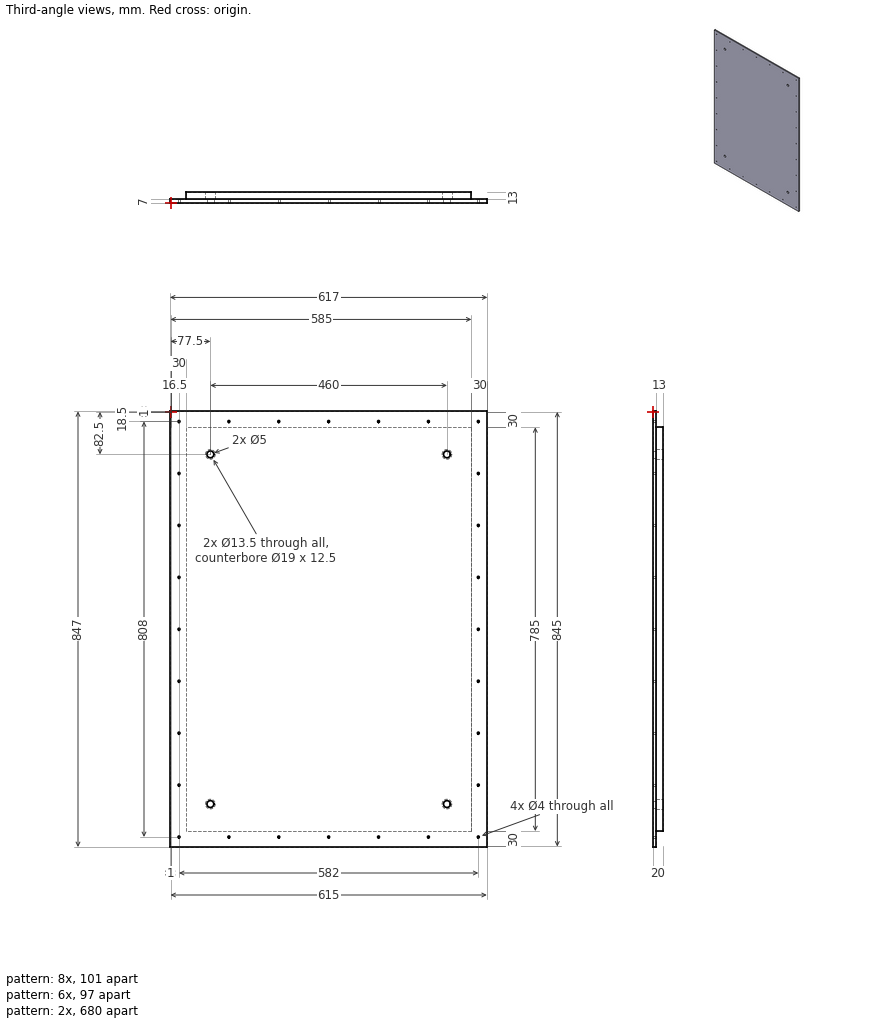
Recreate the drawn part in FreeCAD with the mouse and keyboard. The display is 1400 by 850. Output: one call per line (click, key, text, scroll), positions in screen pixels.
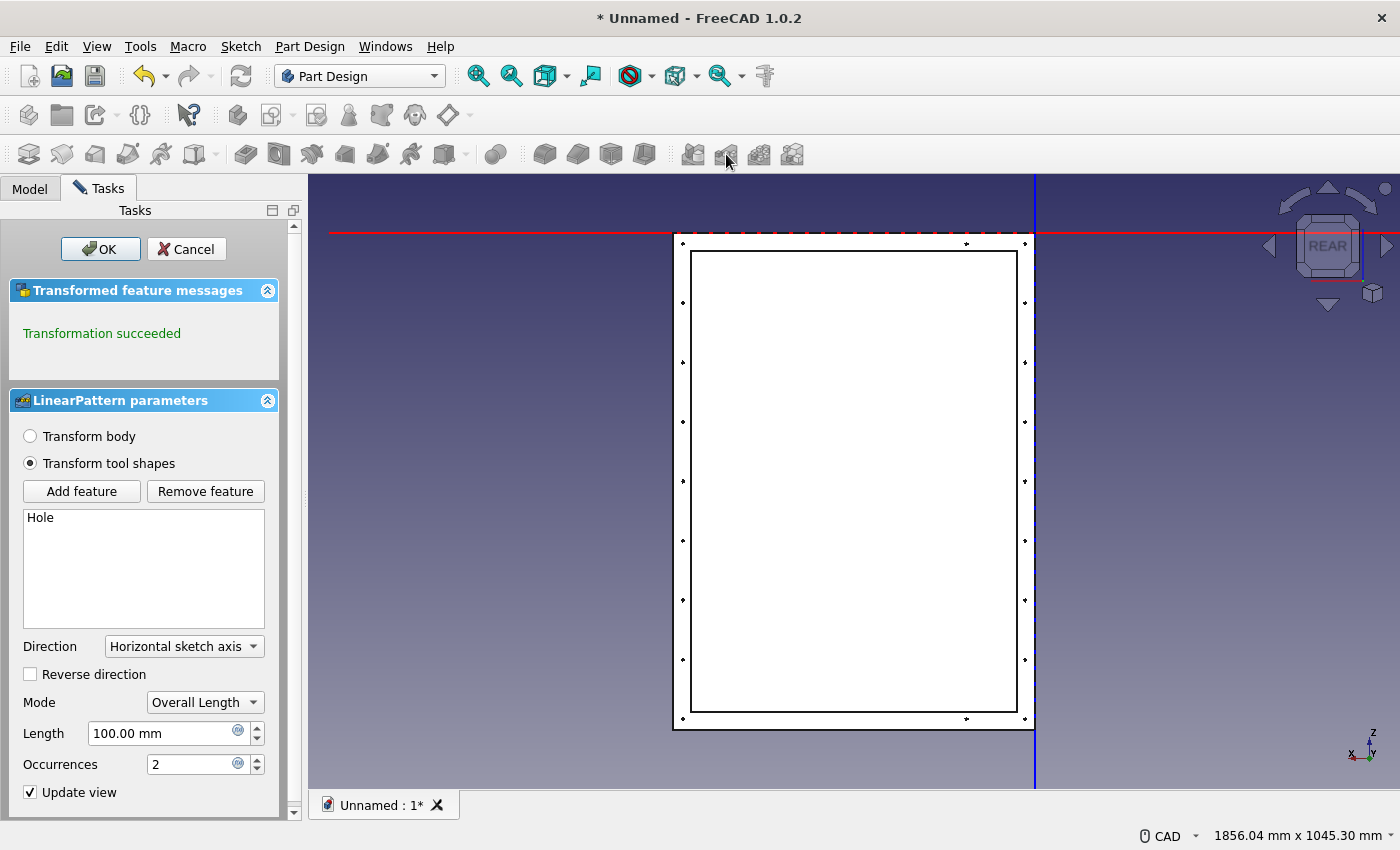
click(185, 646)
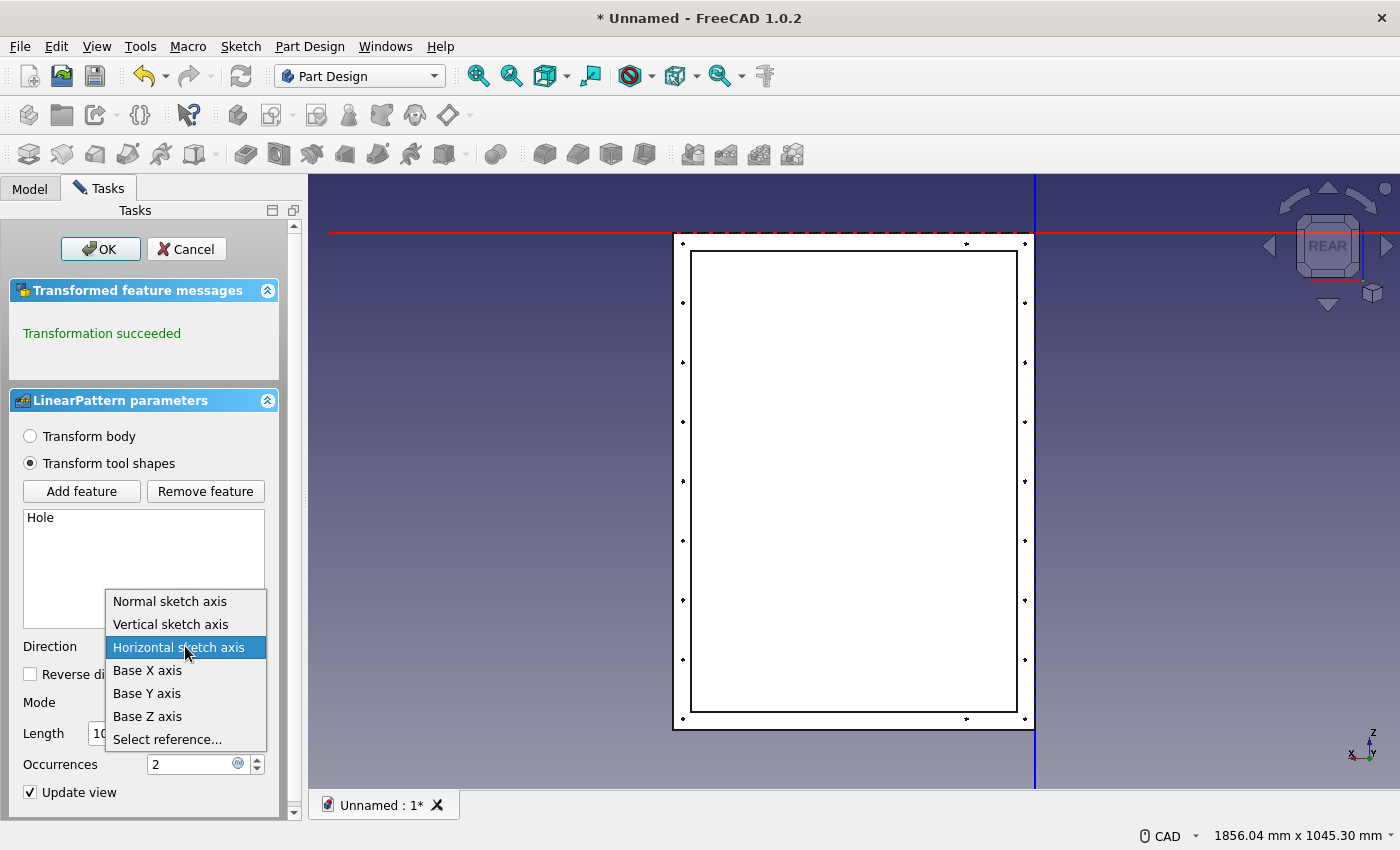
click(184, 670)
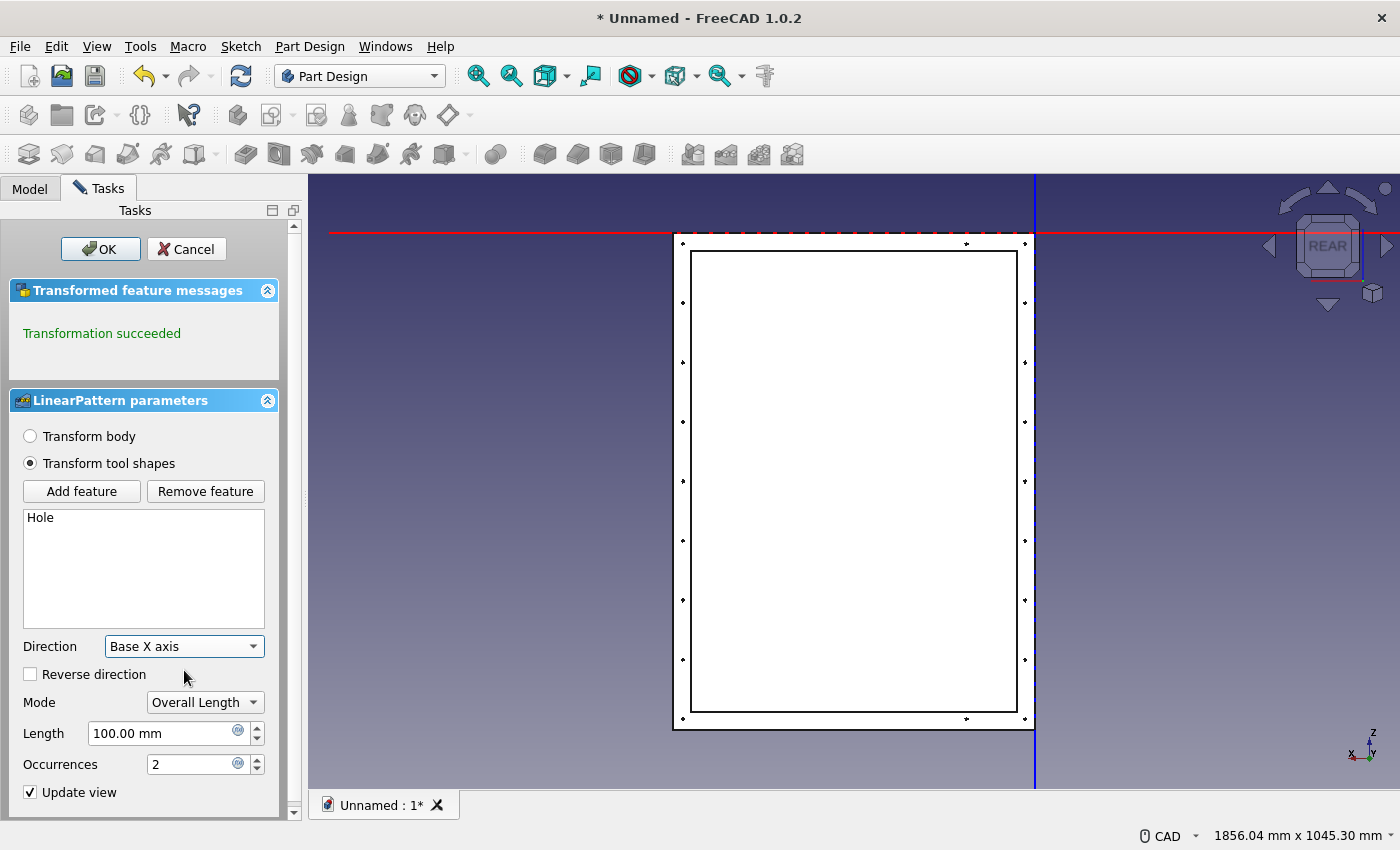
click(206, 702)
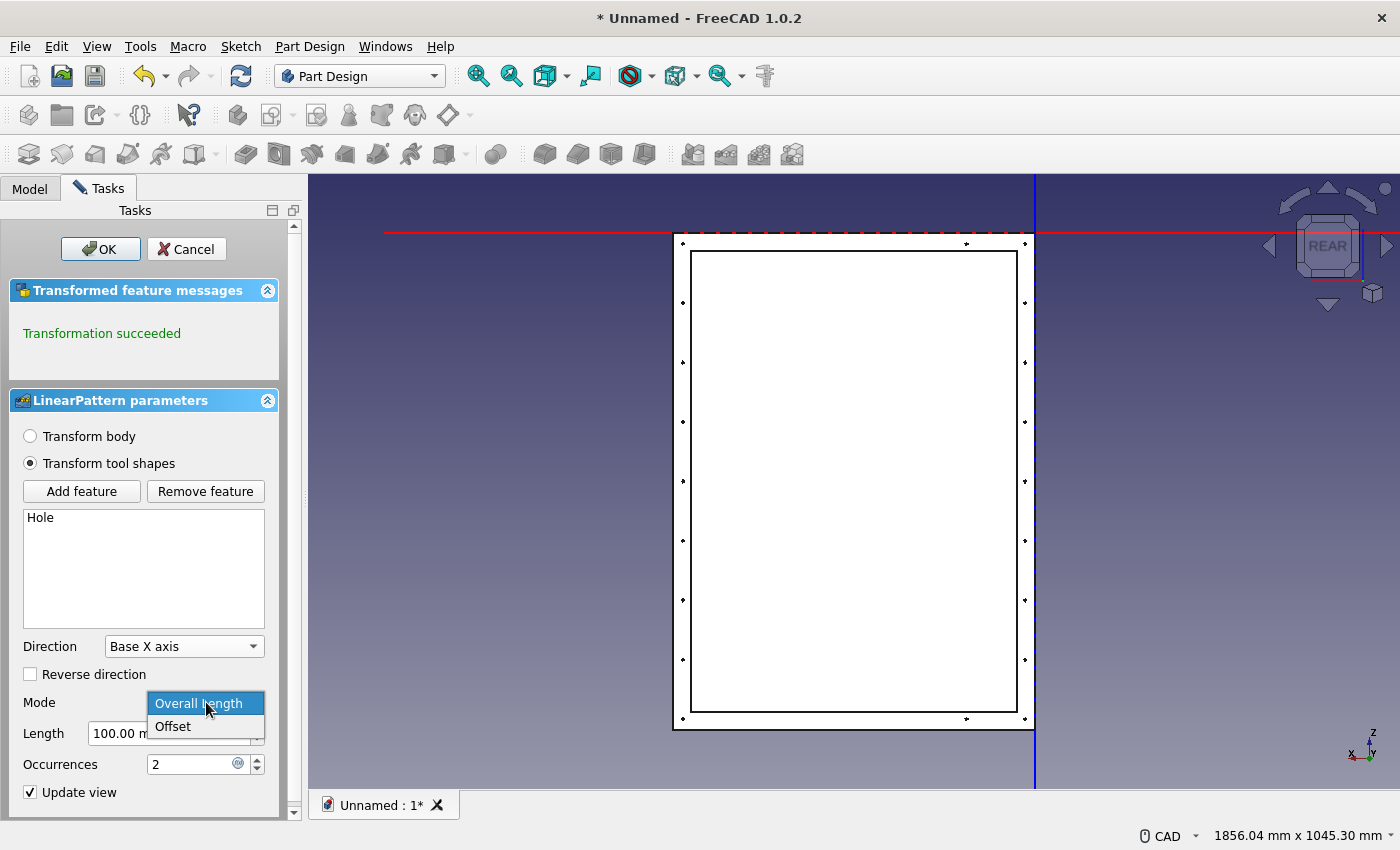
click(204, 726)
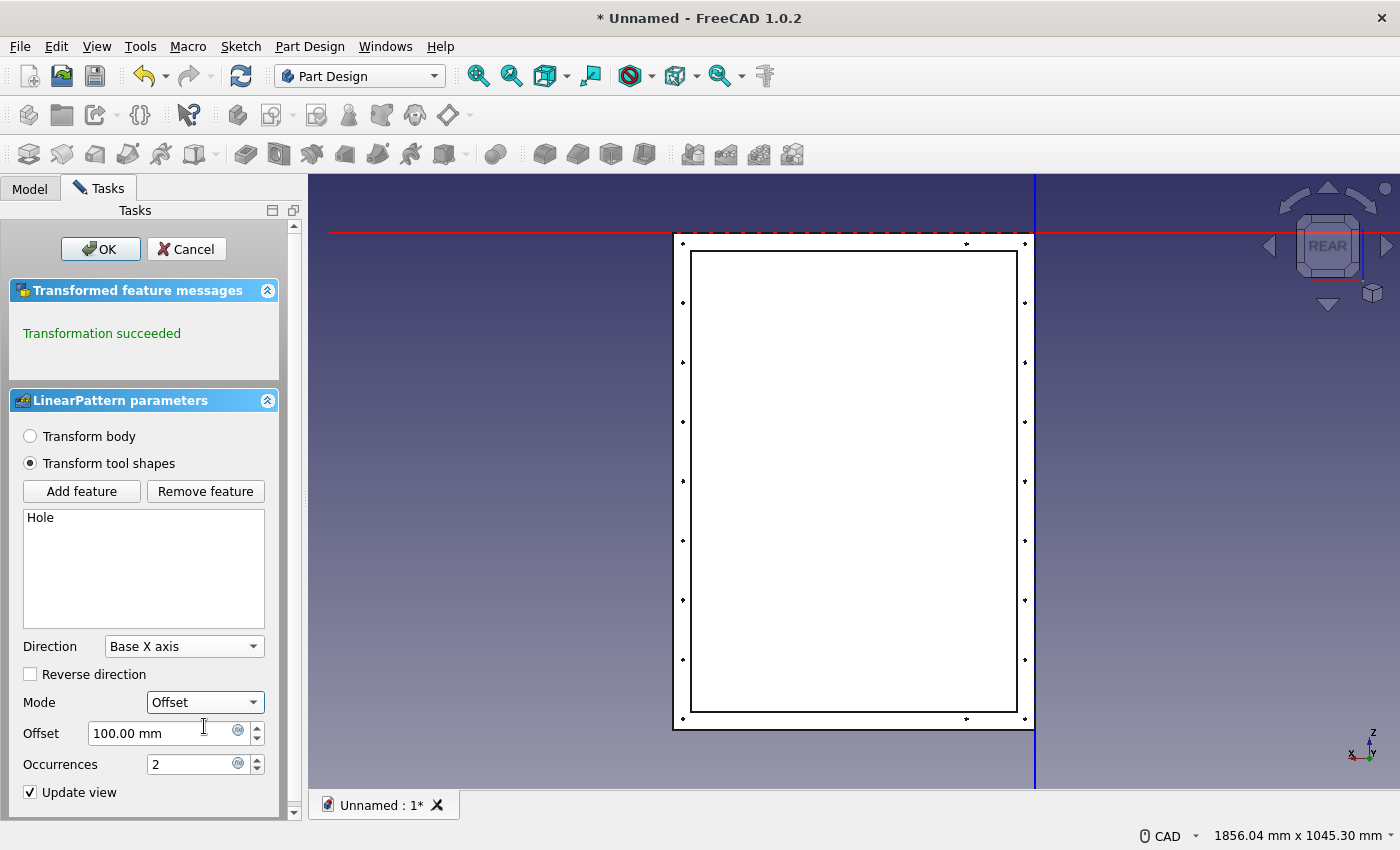
triple_click(170, 734)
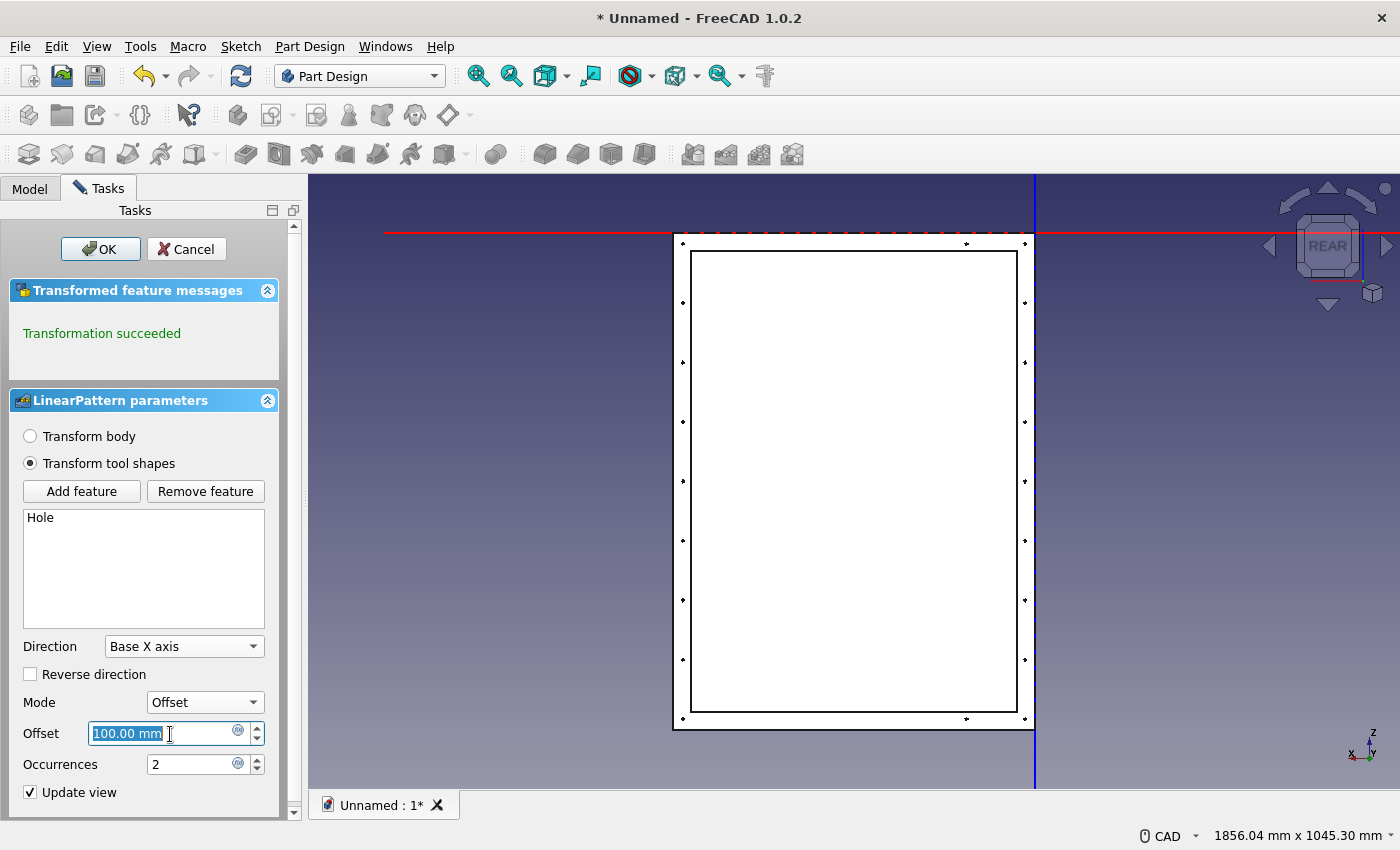
text(97)
key(Tab)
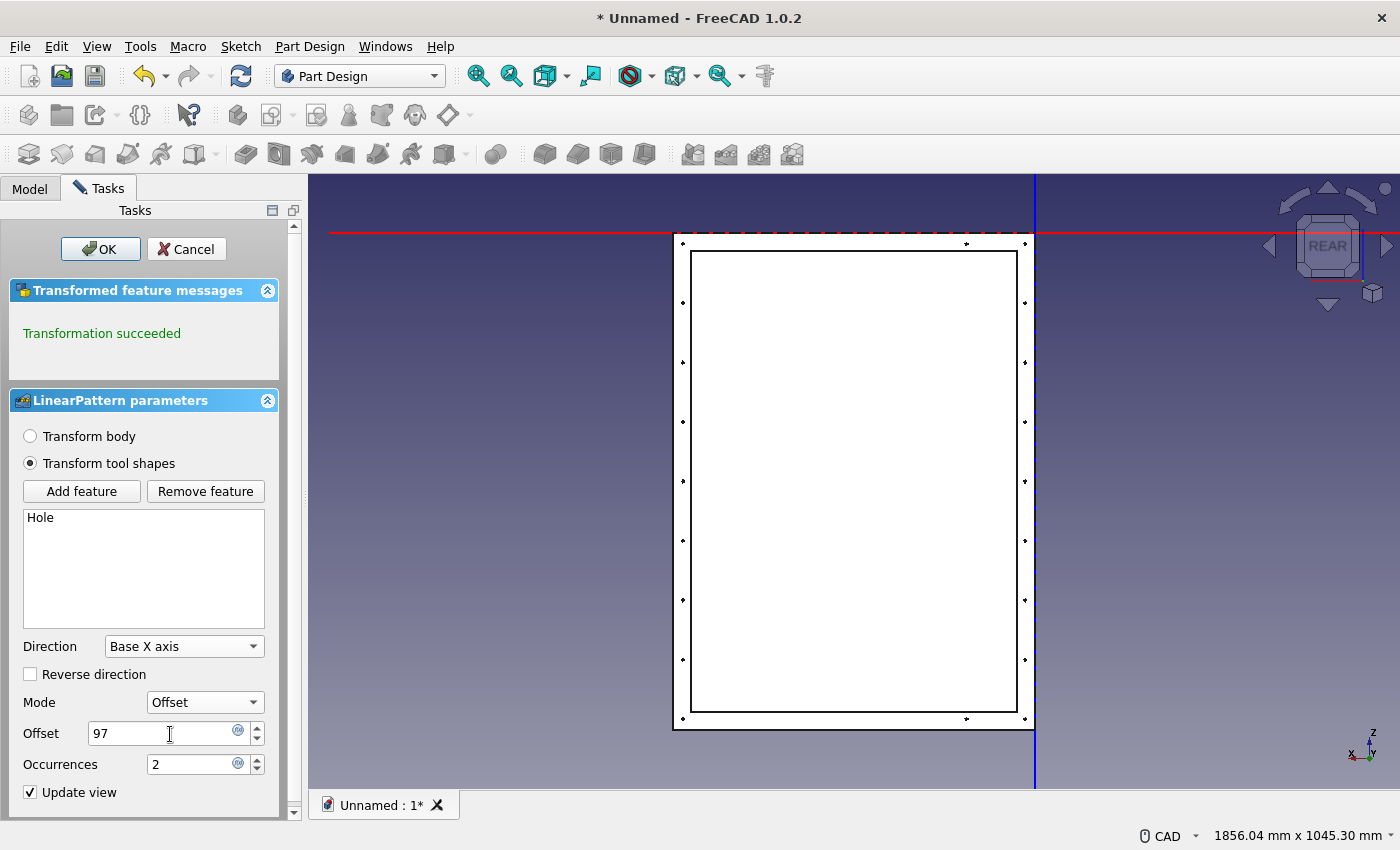
triple_click(199, 764)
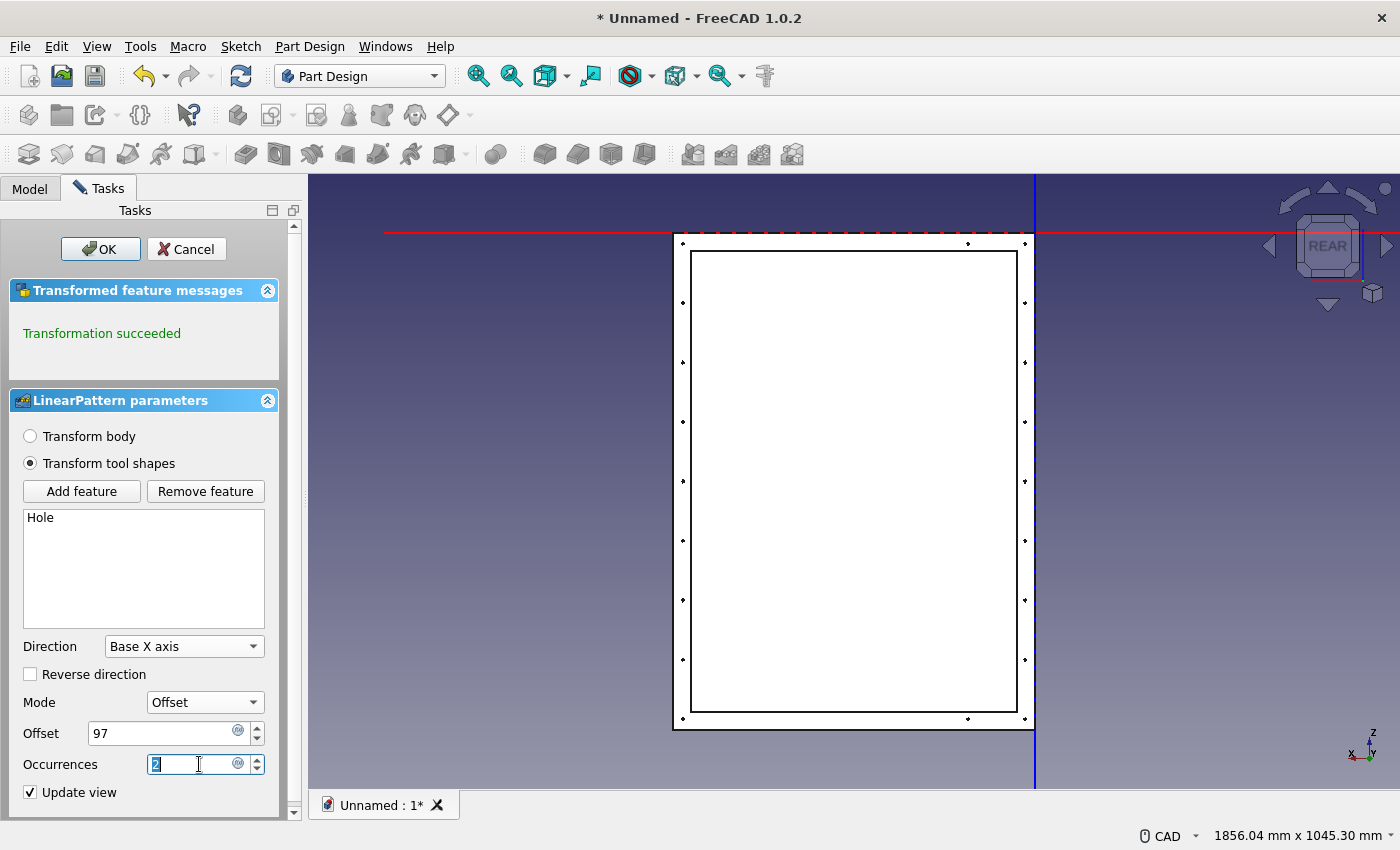
text(6)
key(Tab)